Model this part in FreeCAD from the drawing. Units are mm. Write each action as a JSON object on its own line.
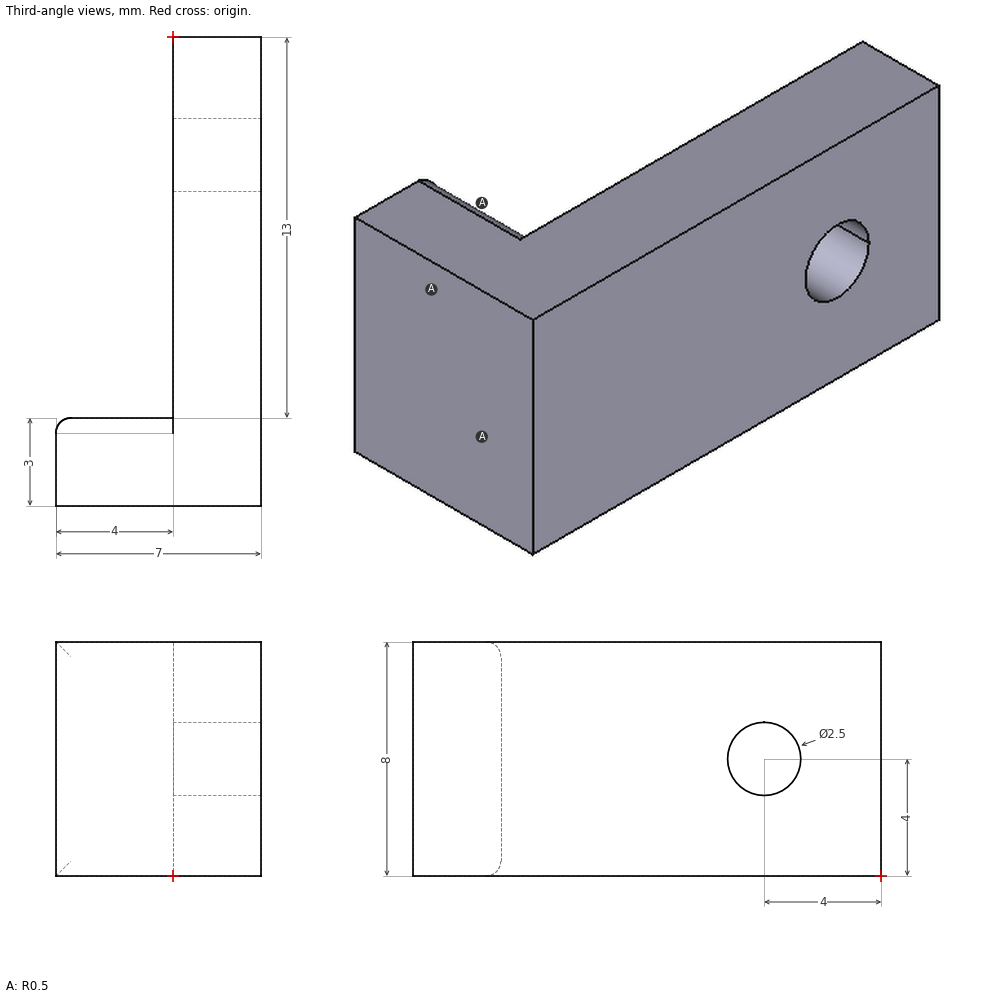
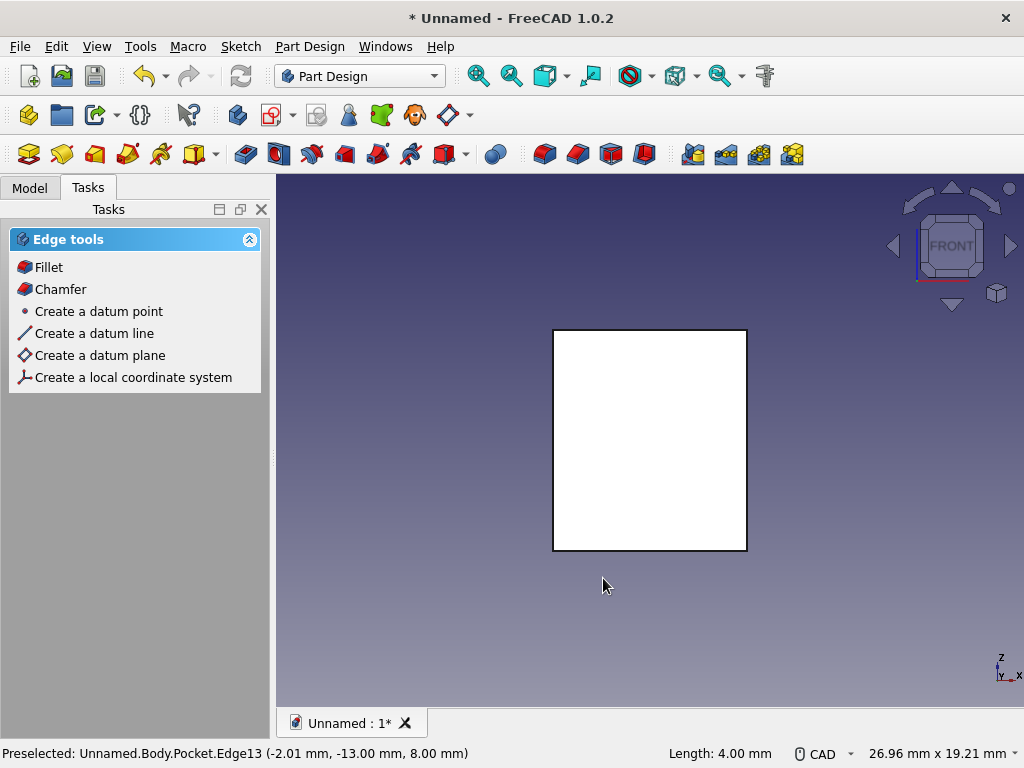
{"action": "key", "text": "3"}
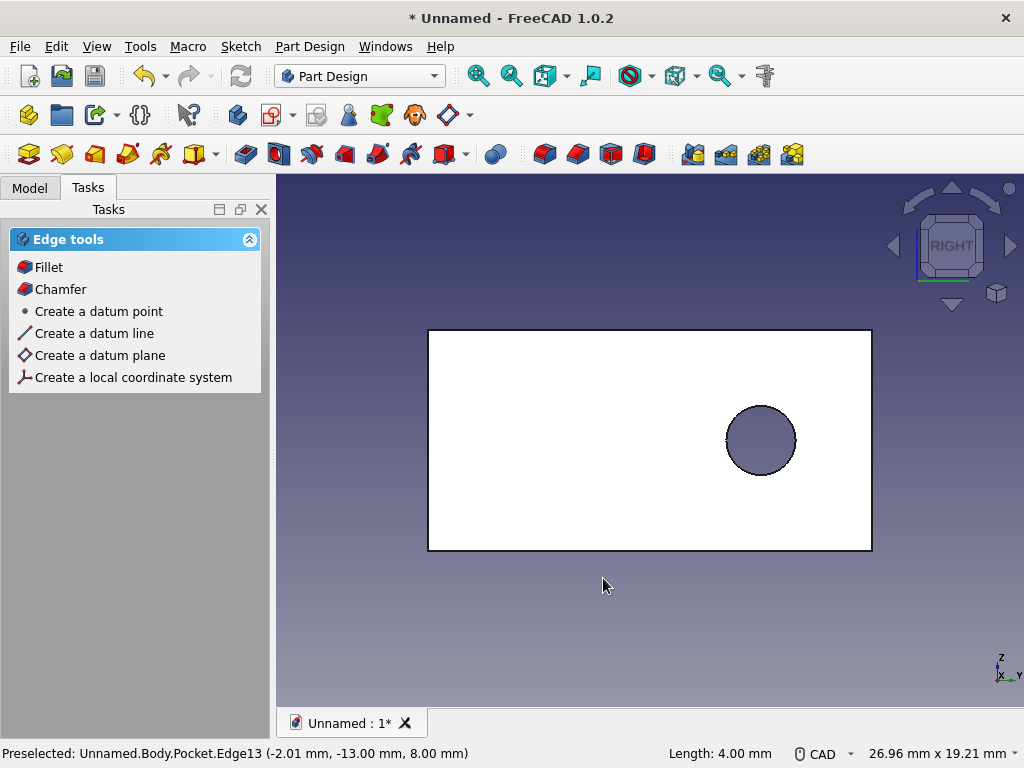
{"action": "key", "text": "5"}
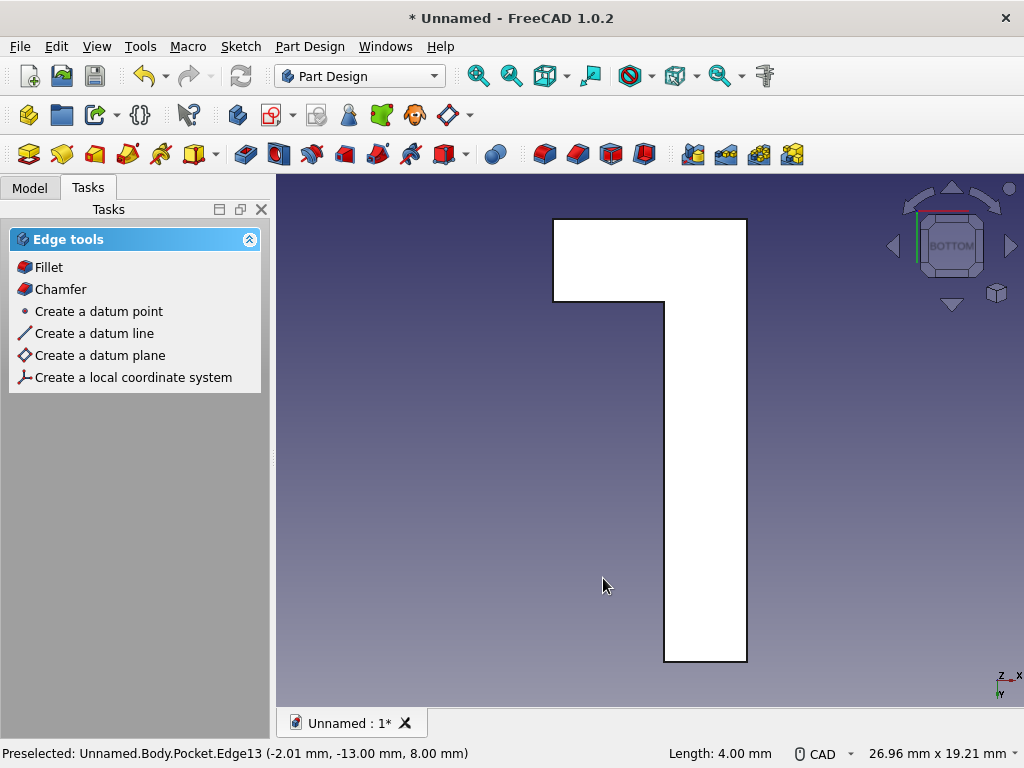
{"action": "left_click", "coordinate": [608, 301], "text": "ctrl"}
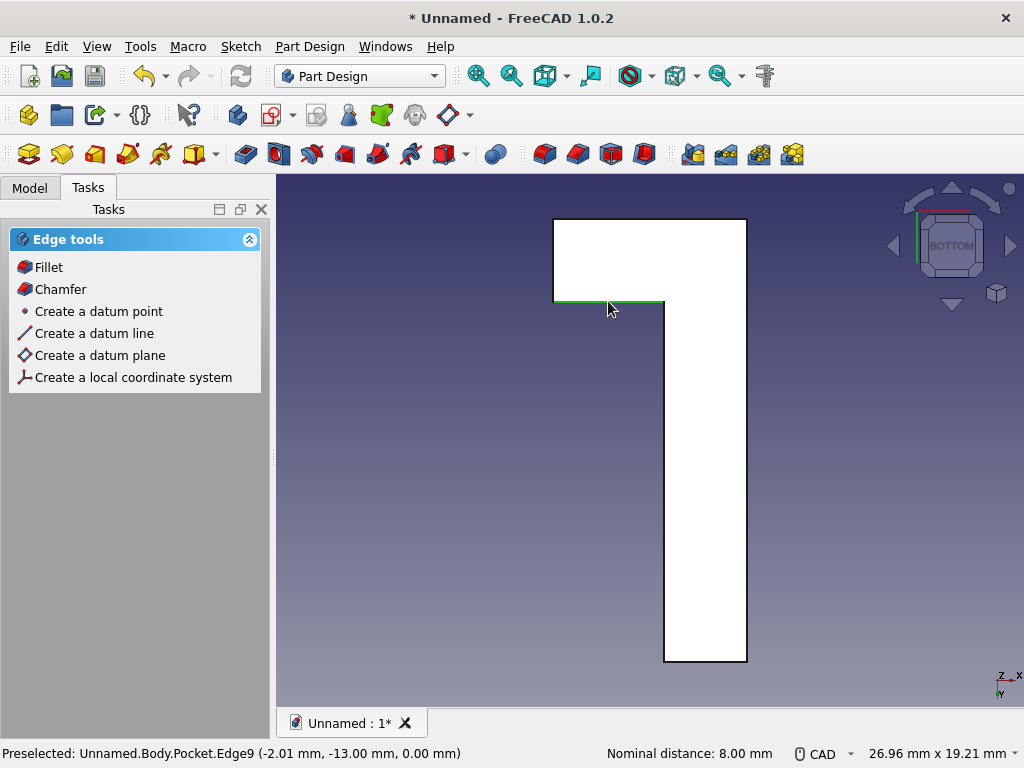
{"action": "key", "text": "4"}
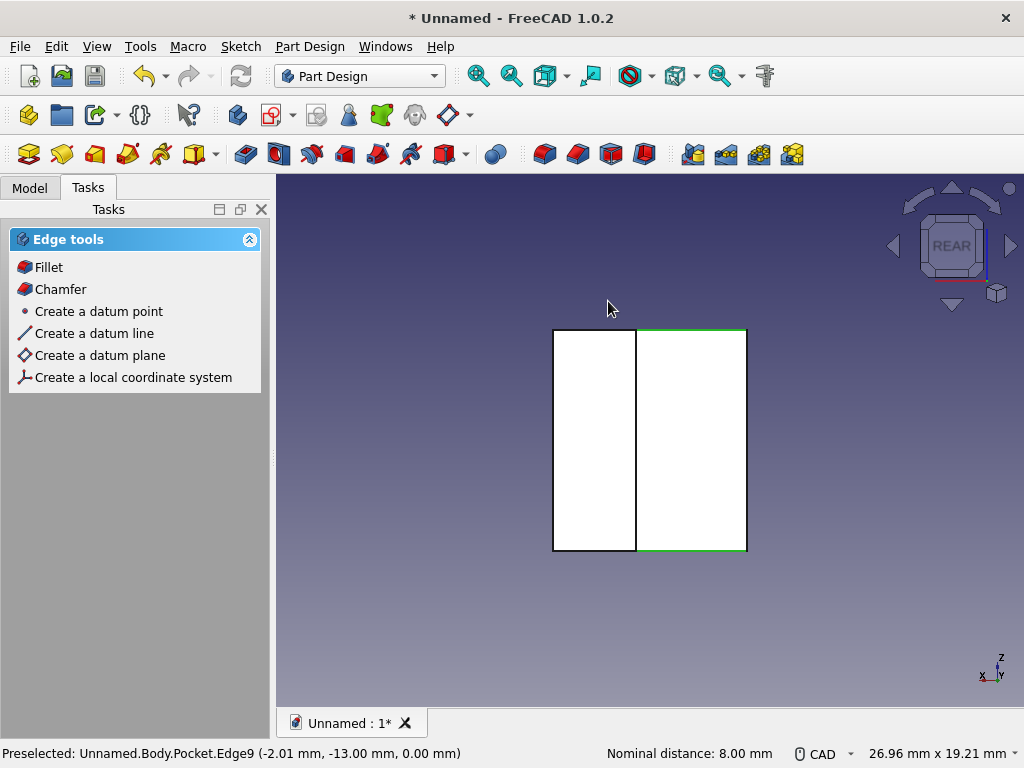
{"action": "left_click", "coordinate": [479, 76]}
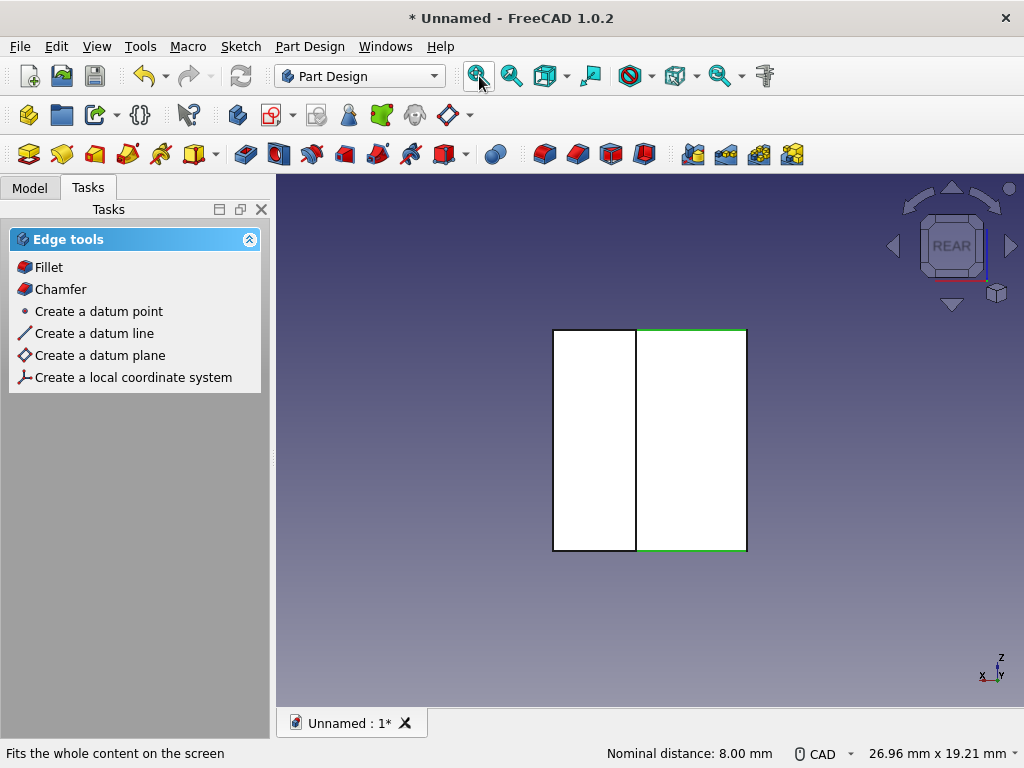
{"action": "left_click", "coordinate": [747, 440], "text": "ctrl"}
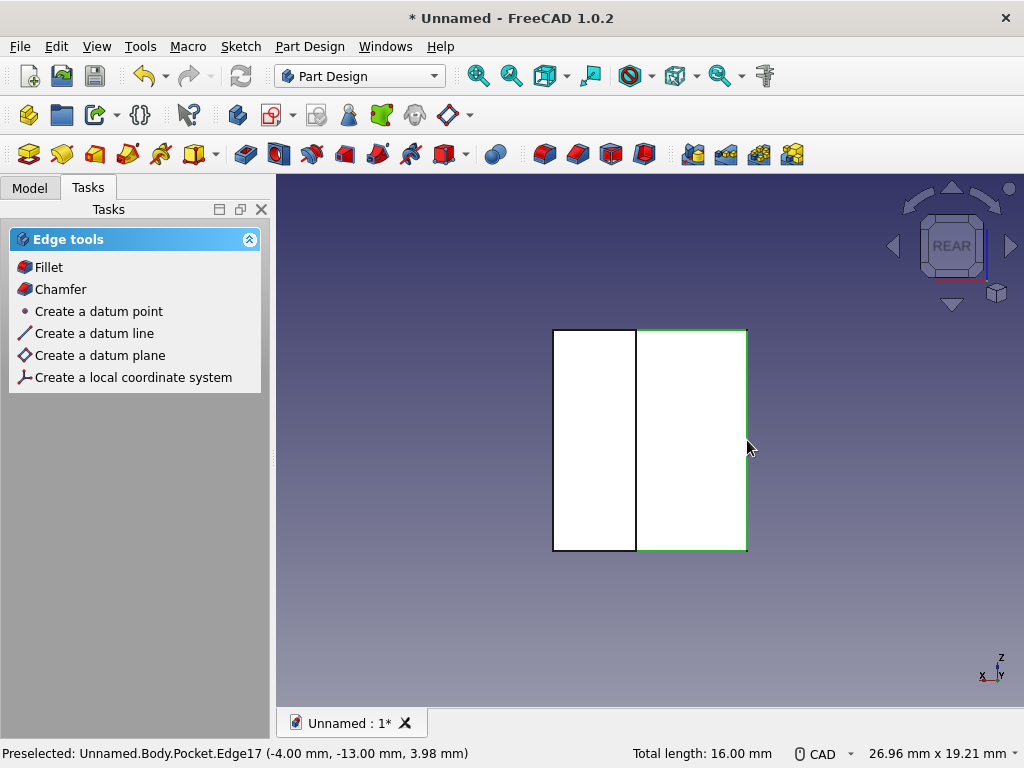
{"action": "left_click", "coordinate": [545, 154]}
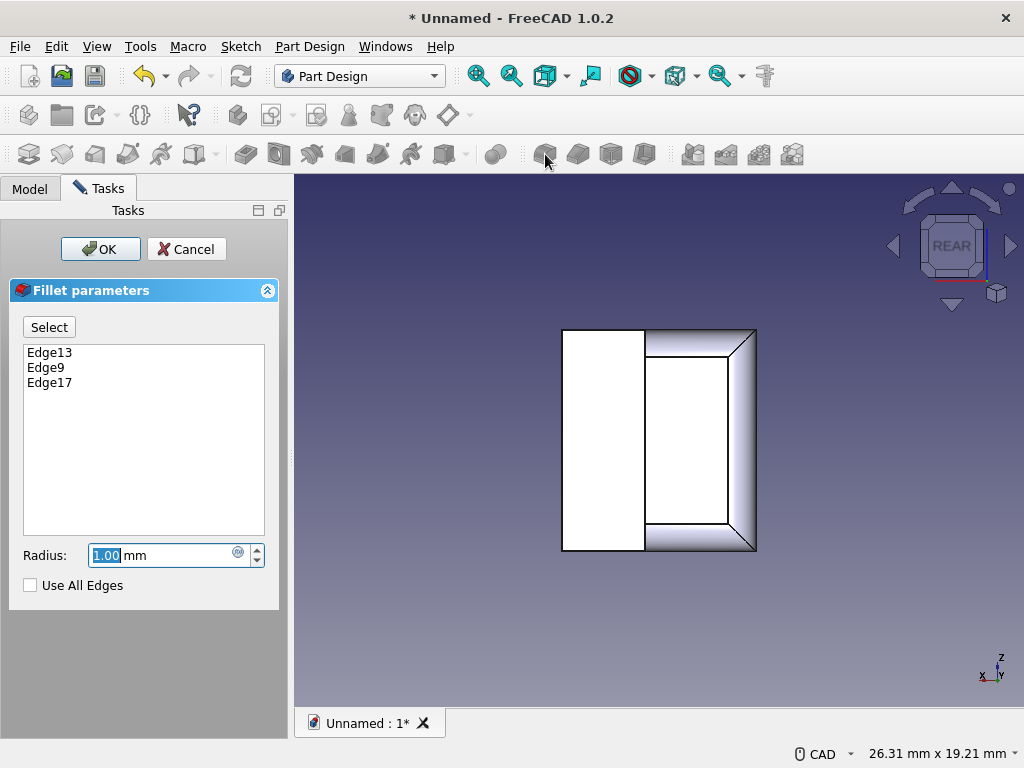
{"action": "type", "text": "0.5"}
{"action": "key", "text": "Tab"}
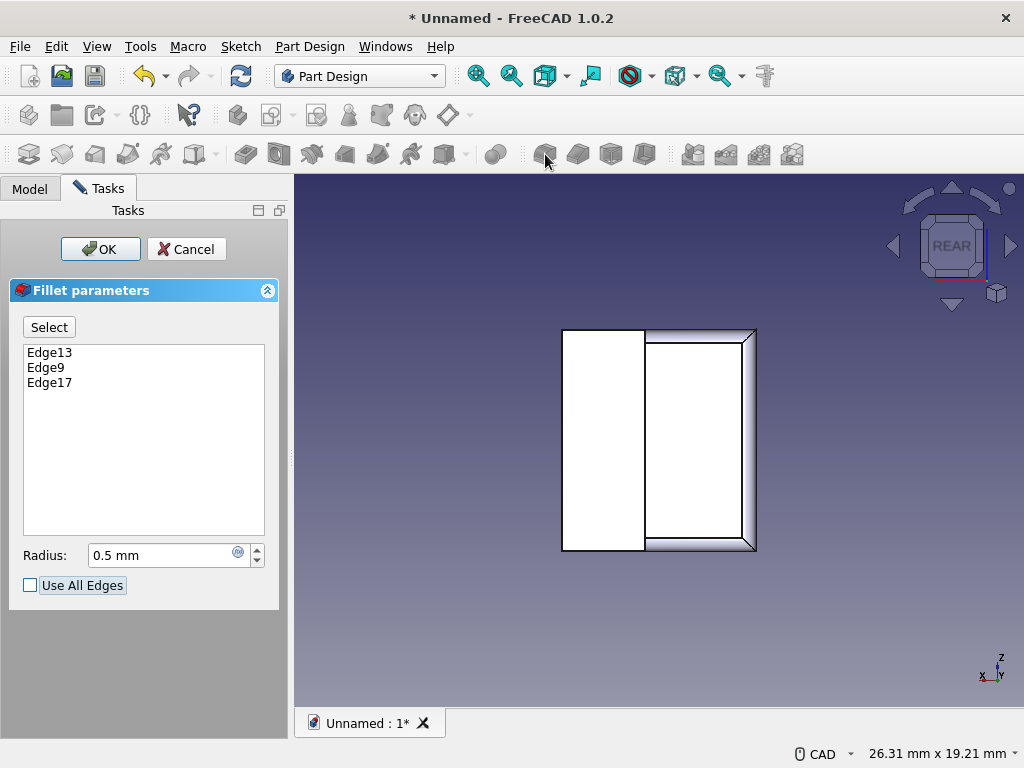
{"action": "left_click", "coordinate": [101, 249]}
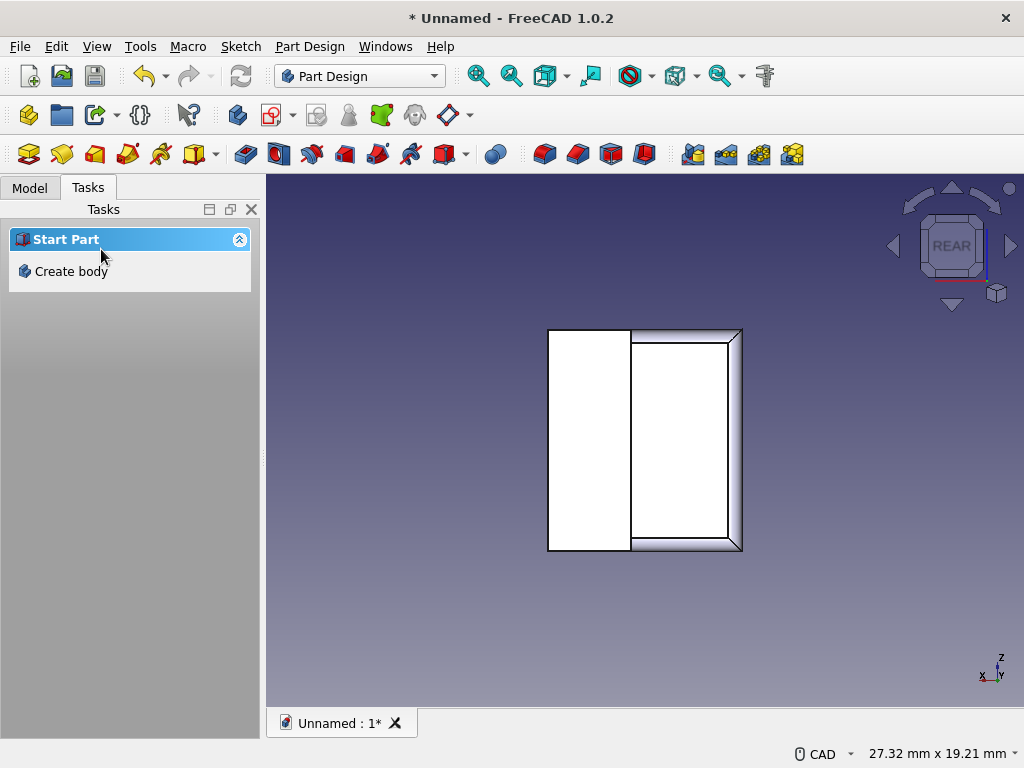
{"action": "key", "text": "0"}